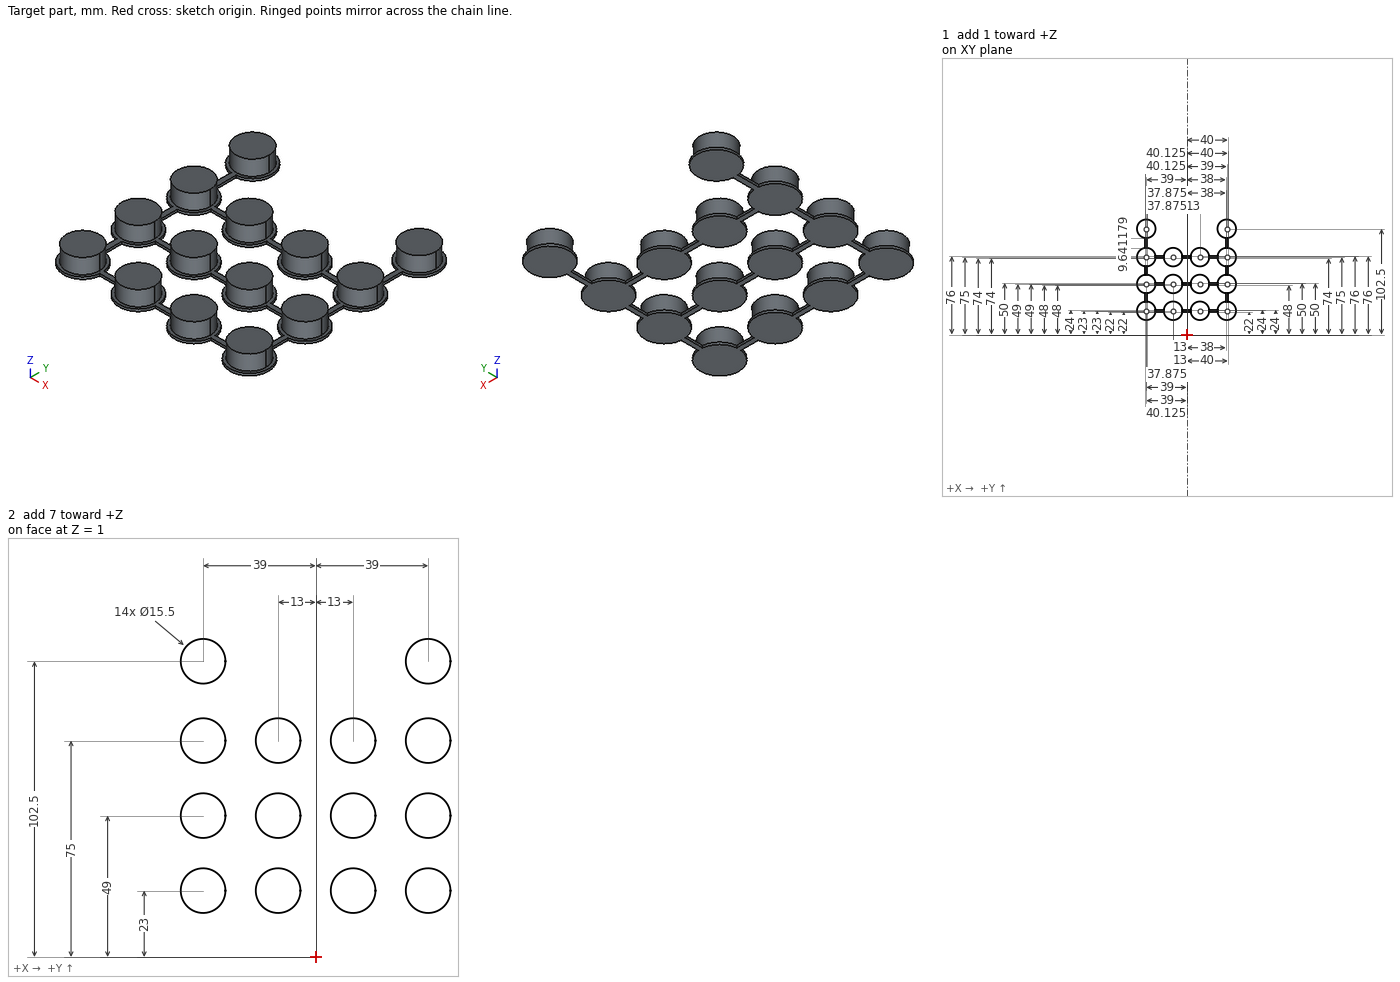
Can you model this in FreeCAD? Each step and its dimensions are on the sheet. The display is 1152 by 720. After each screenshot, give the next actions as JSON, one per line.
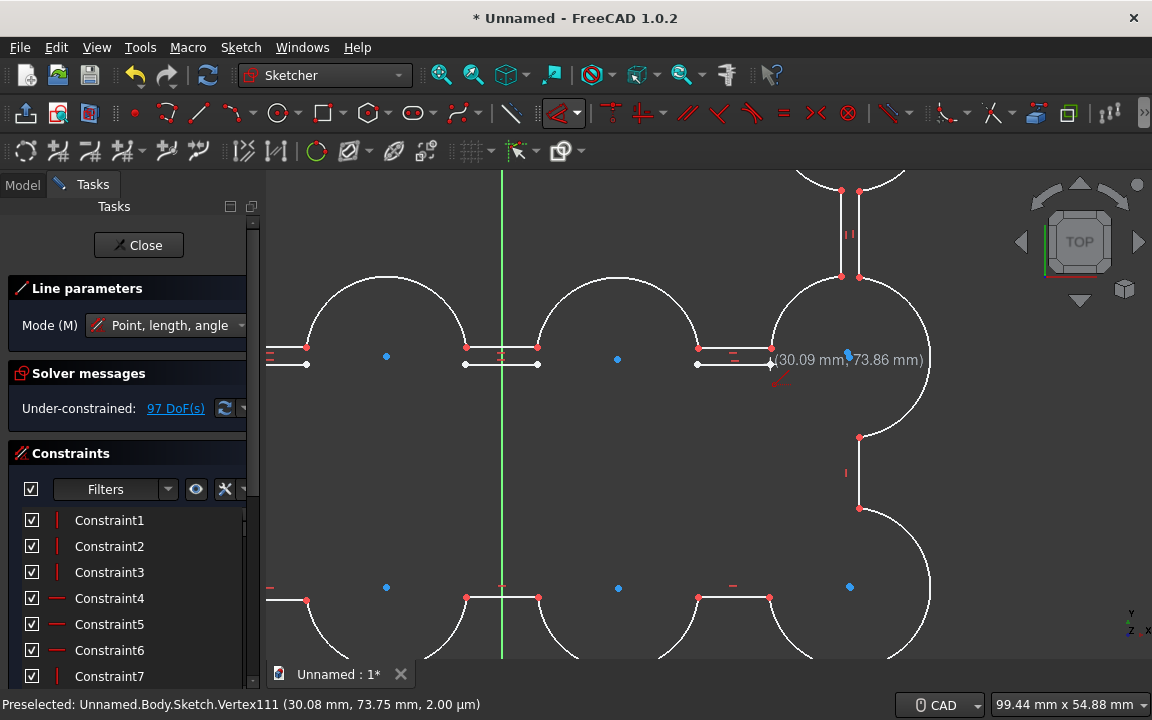
{"action": "left_click", "coordinate": [841, 435]}
{"action": "left_click", "coordinate": [841, 507]}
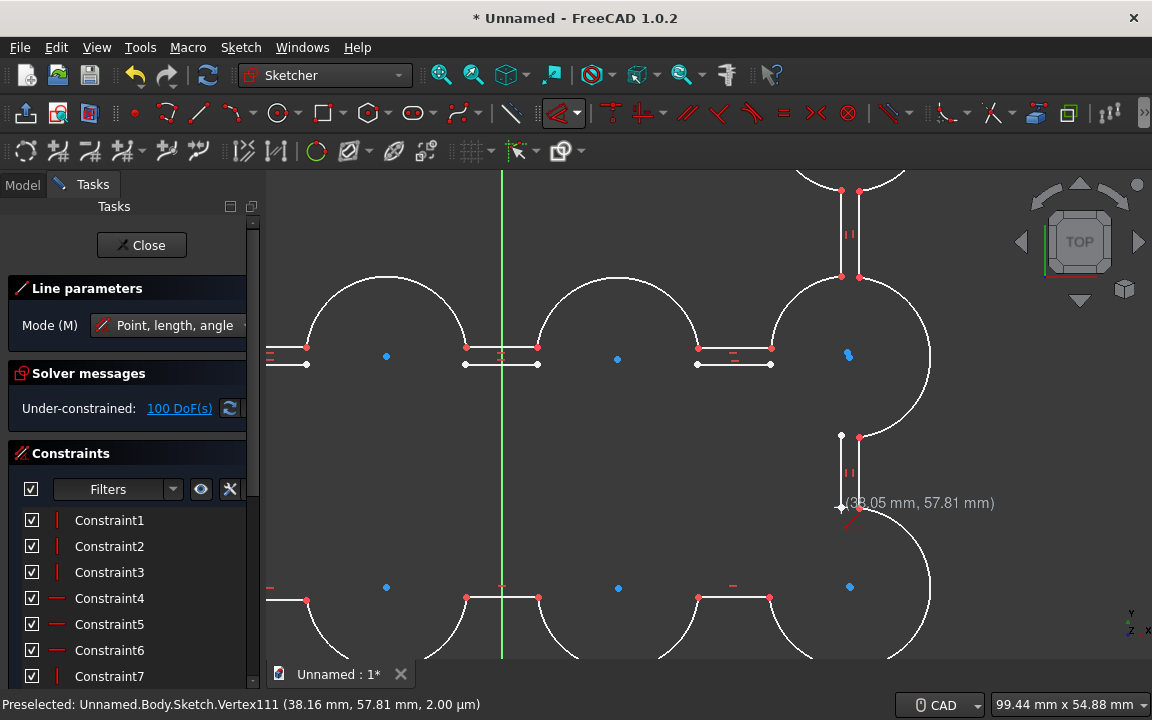
{"action": "left_click", "coordinate": [770, 578]}
{"action": "left_click", "coordinate": [697, 578]}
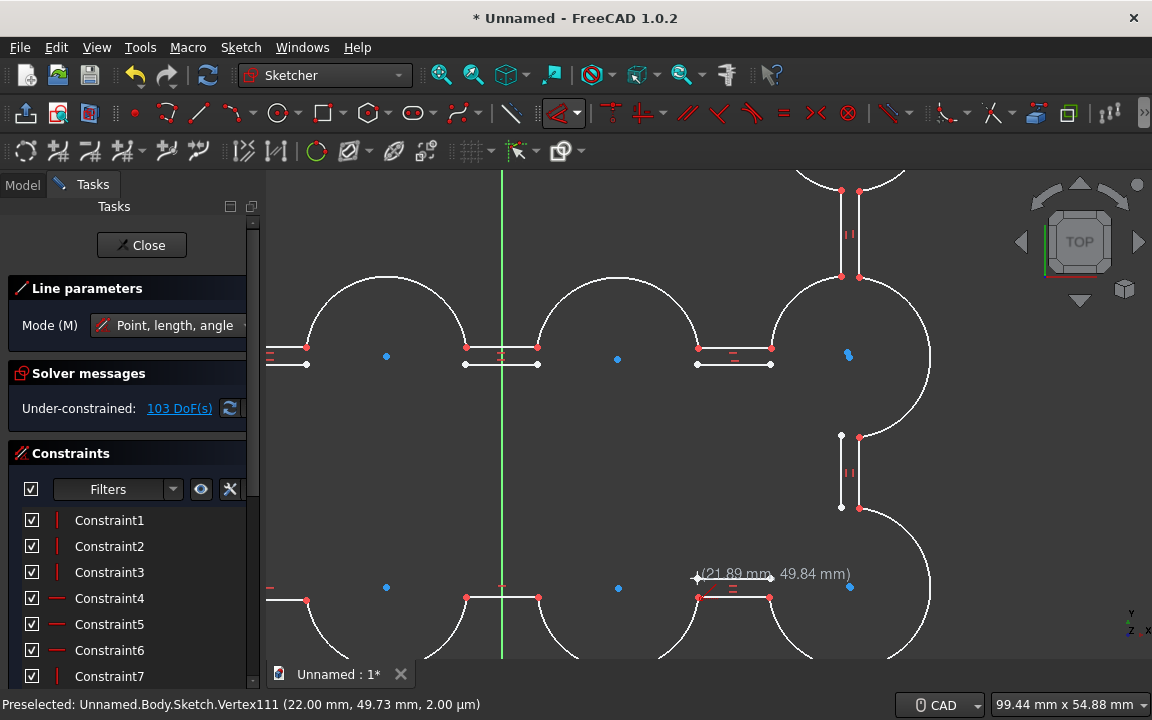
{"action": "left_click", "coordinate": [538, 578]}
{"action": "left_click", "coordinate": [466, 578]}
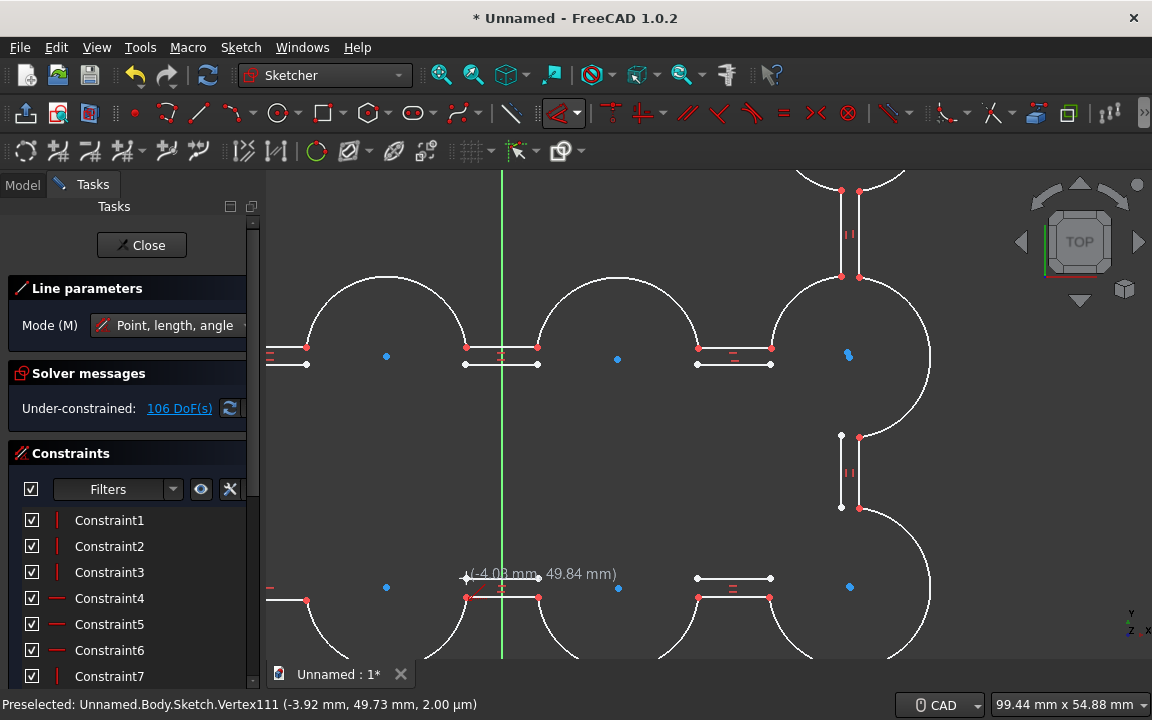
{"action": "left_click", "coordinate": [306, 578]}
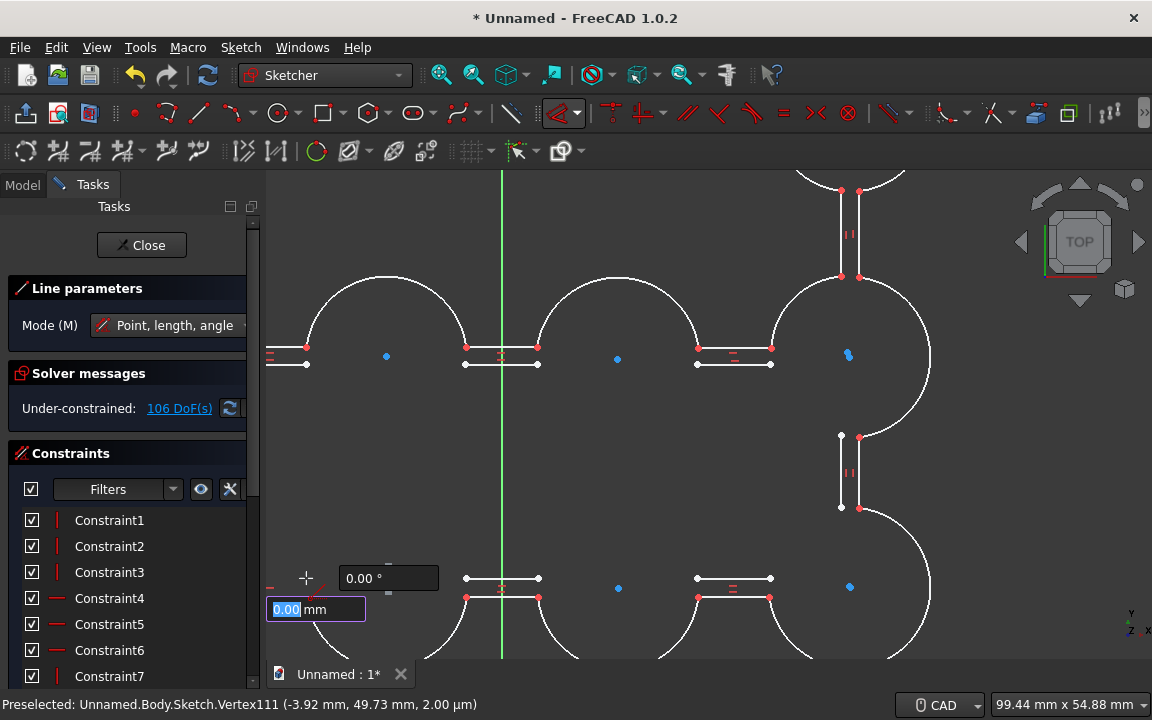
{"action": "scroll", "coordinate": [700, 366], "scroll_direction": "down", "scroll_amount": 6}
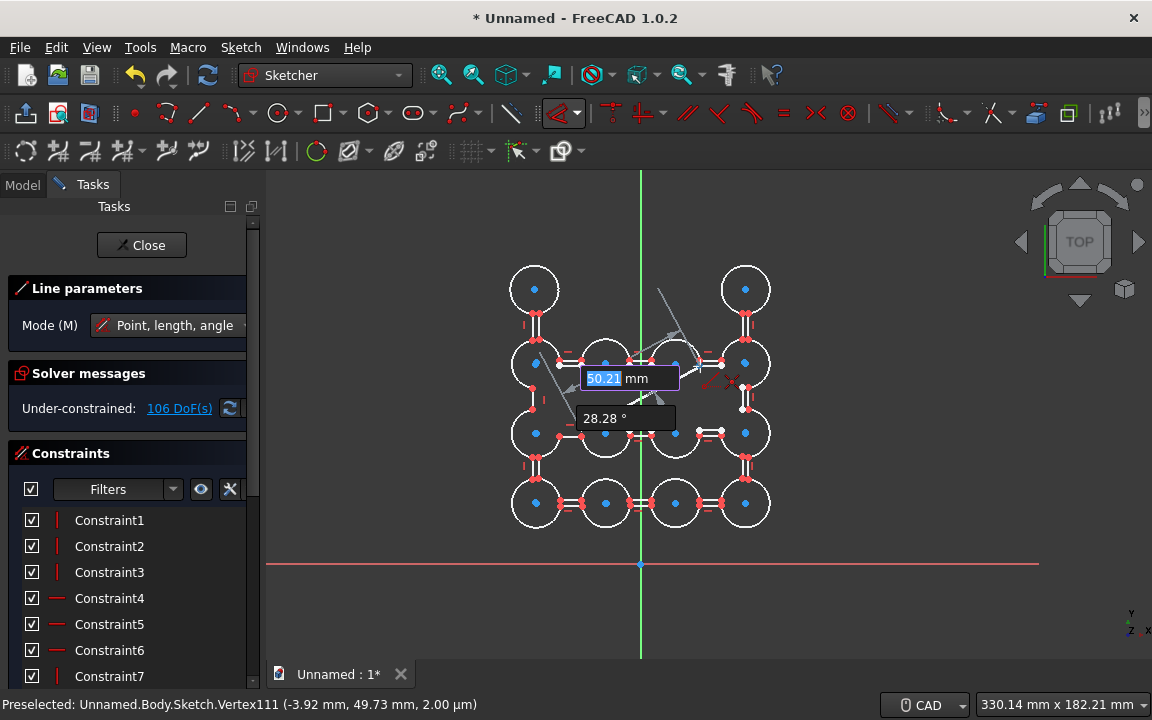
{"action": "scroll", "coordinate": [560, 430], "scroll_direction": "up", "scroll_amount": 6}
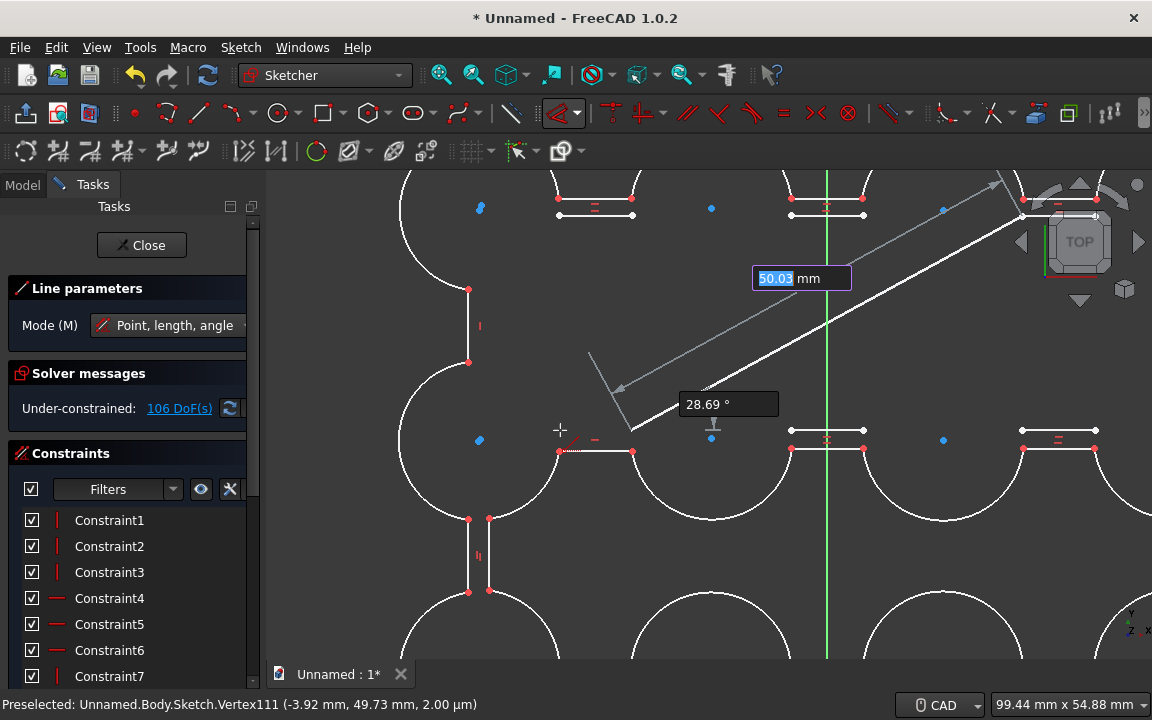
{"action": "left_click", "coordinate": [559, 429]}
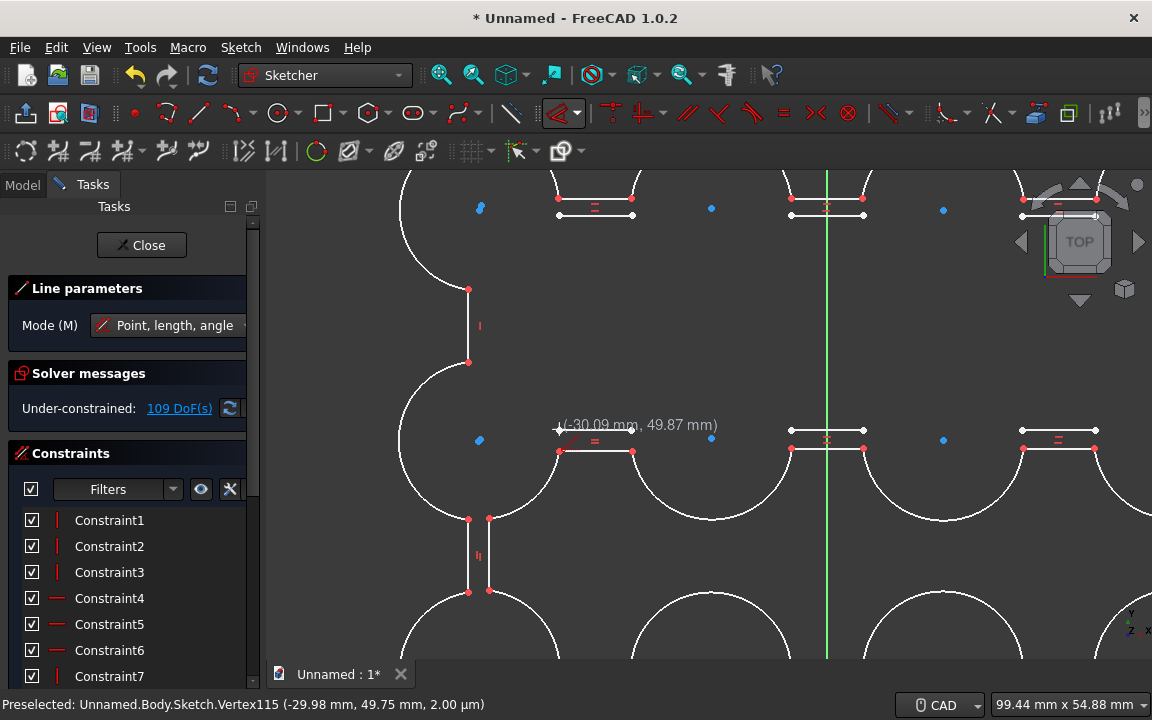
{"action": "left_click", "coordinate": [490, 358]}
{"action": "left_click", "coordinate": [490, 286]}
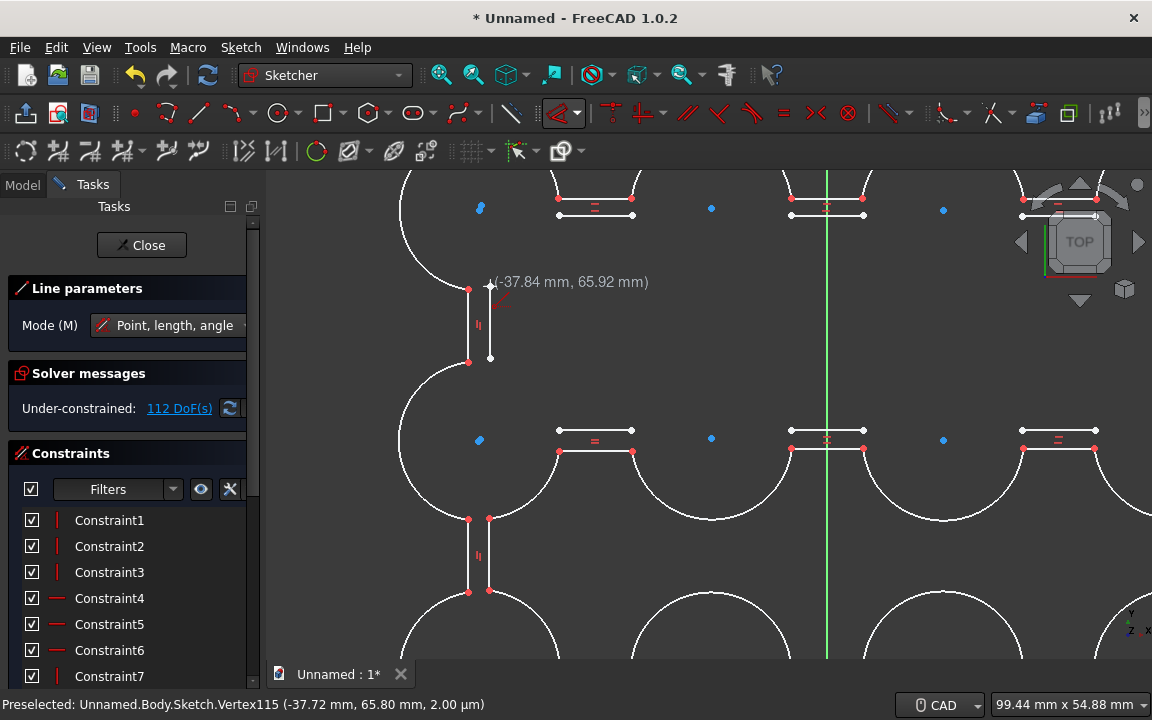
{"action": "left_click", "coordinate": [232, 114]}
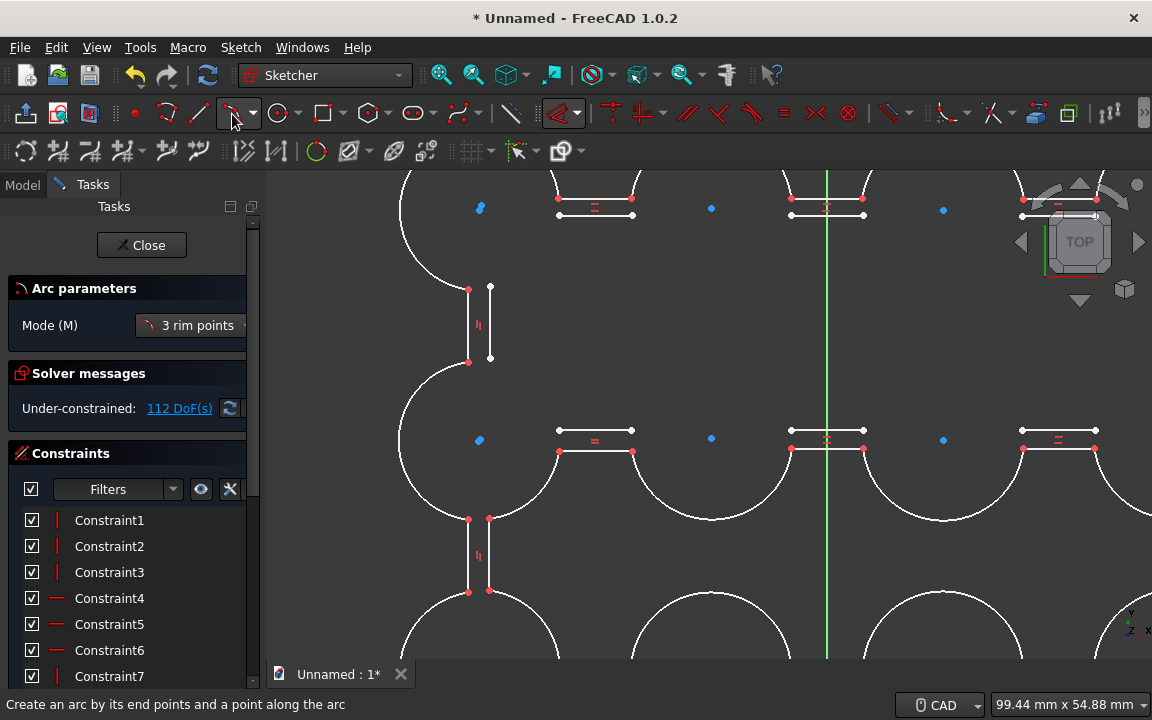
{"action": "left_click", "coordinate": [632, 216]}
{"action": "left_click", "coordinate": [791, 216]}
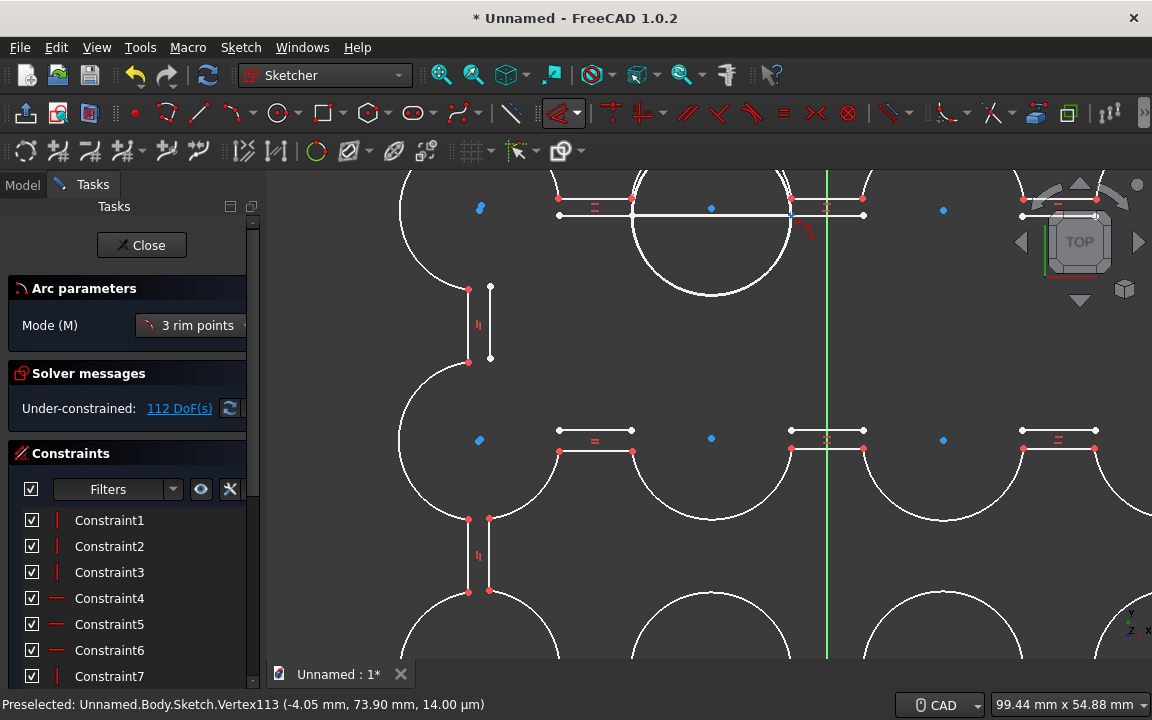
{"action": "scroll", "coordinate": [560, 430], "scroll_direction": "down", "scroll_amount": 6}